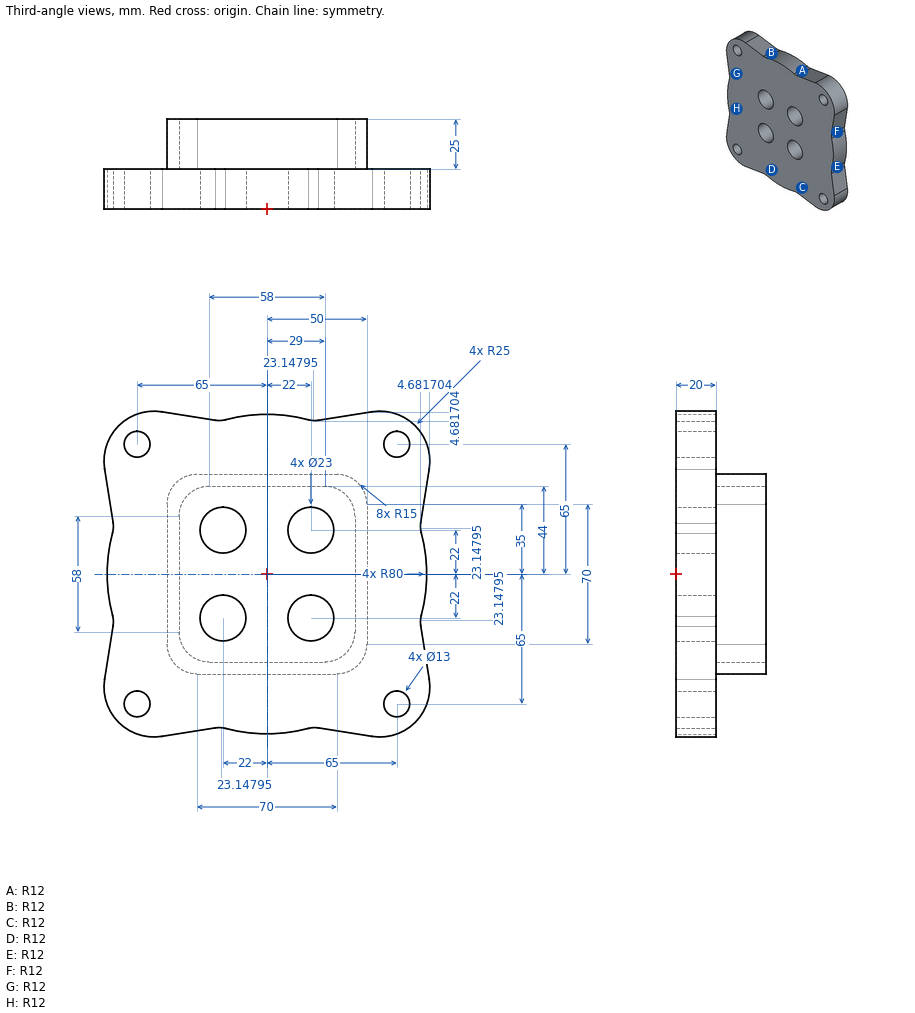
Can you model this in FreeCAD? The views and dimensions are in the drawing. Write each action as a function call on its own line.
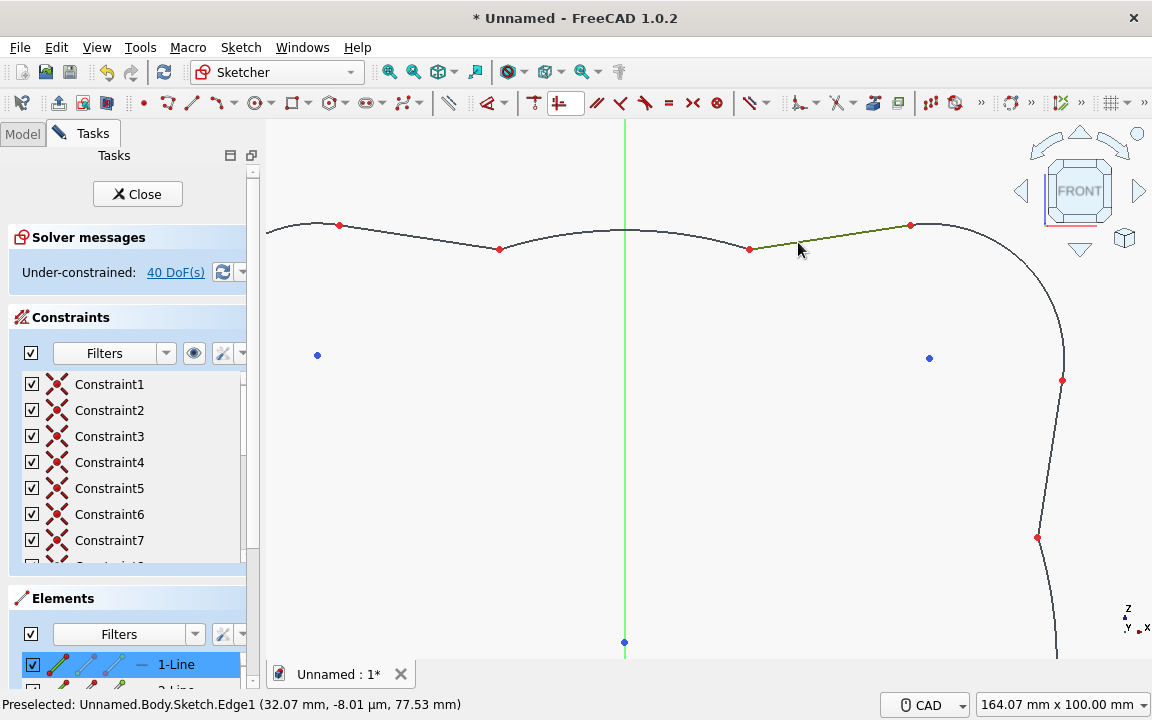
click(984, 236)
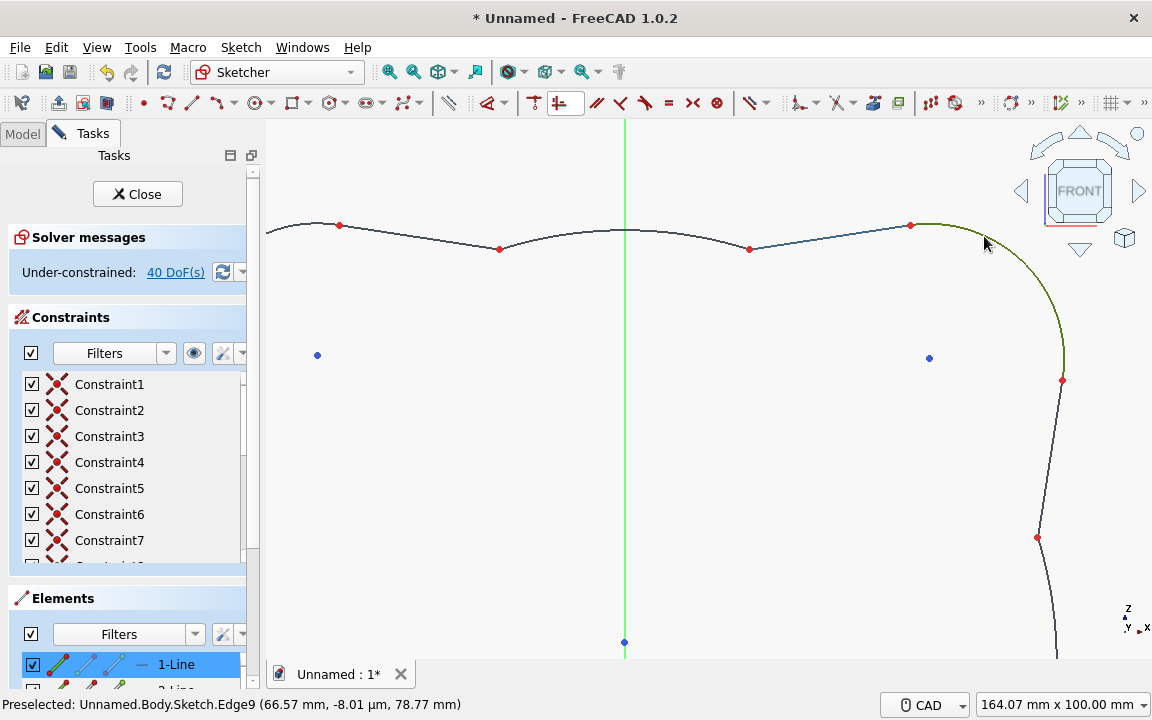
click(646, 104)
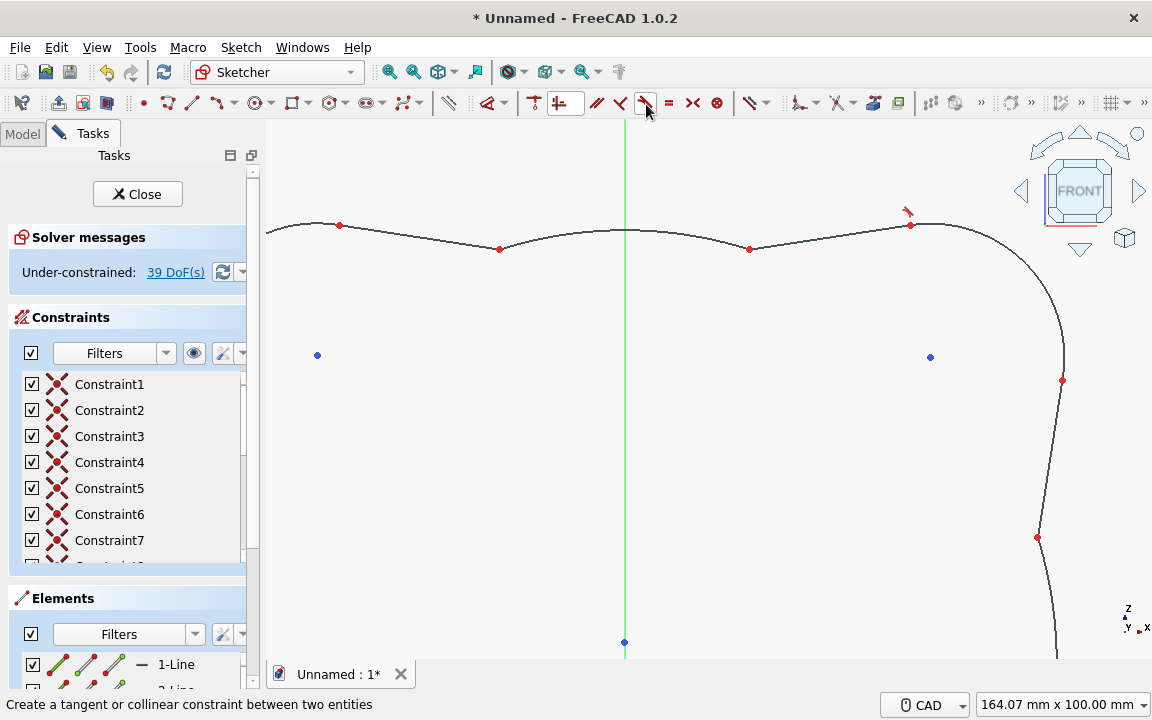
scroll(650, 231, down, 5)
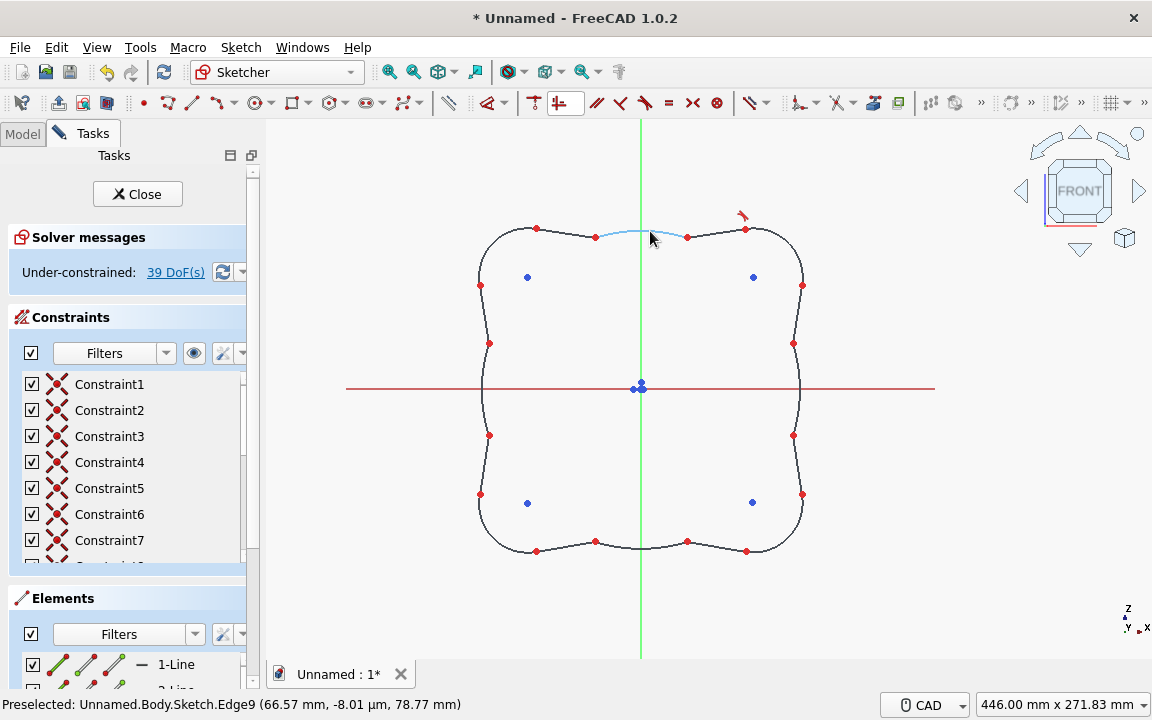
click(799, 303)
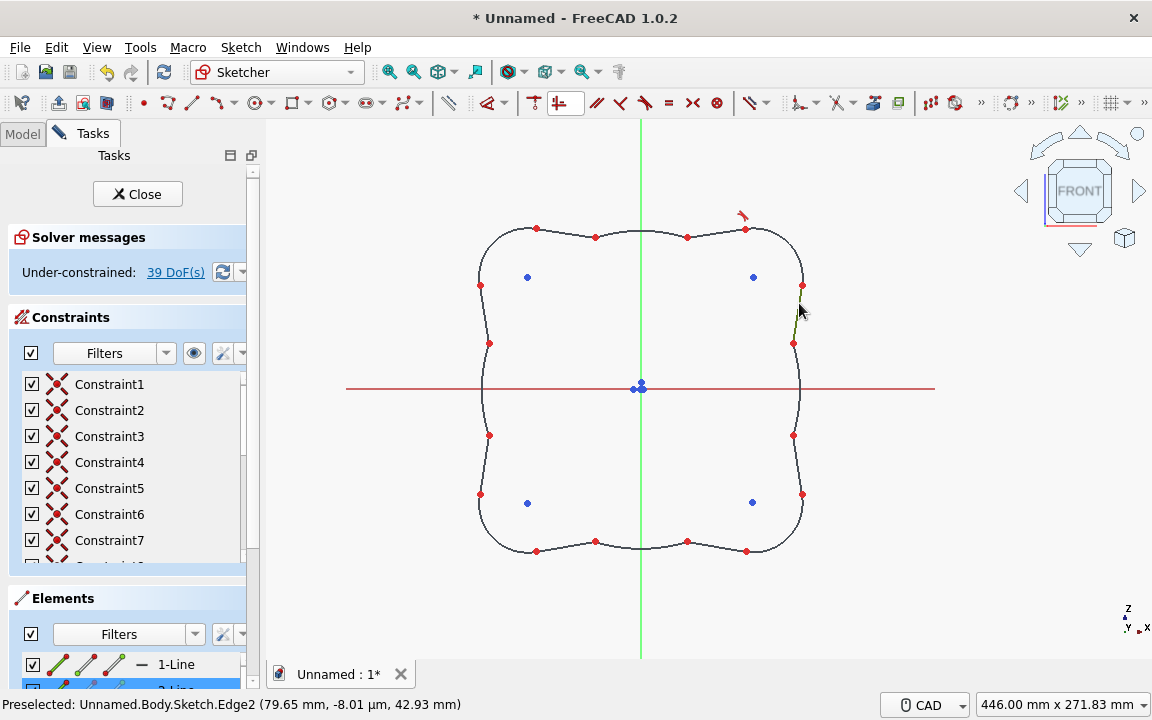
click(799, 259)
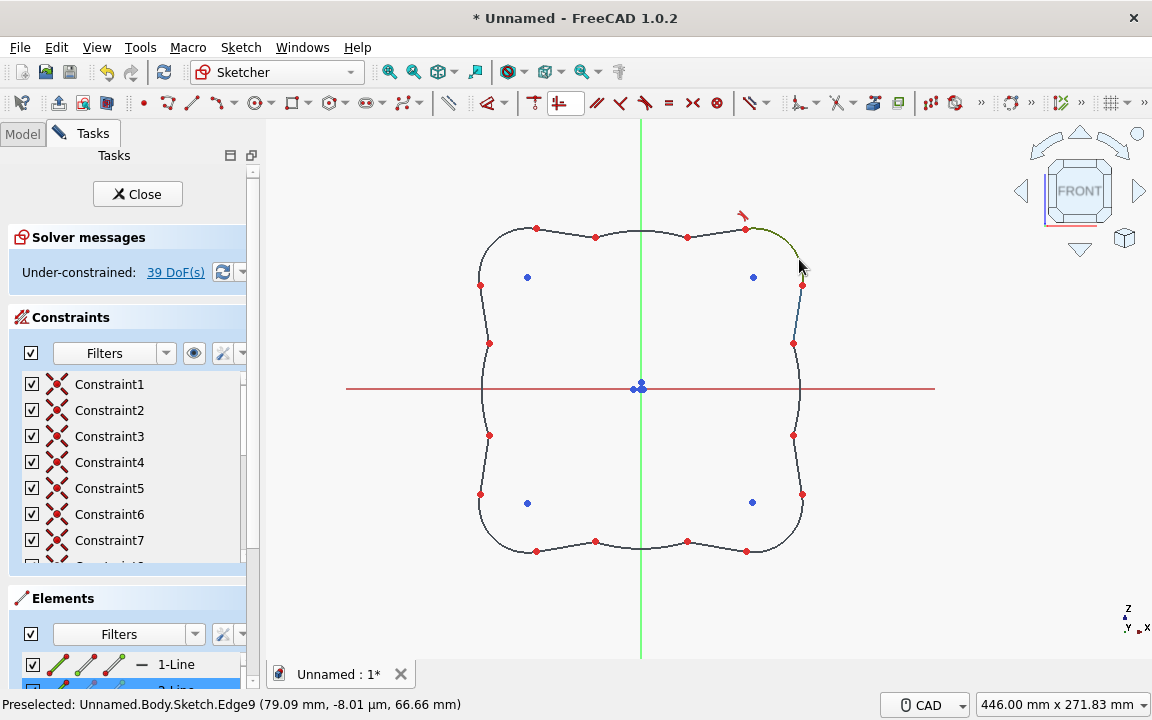
click(646, 104)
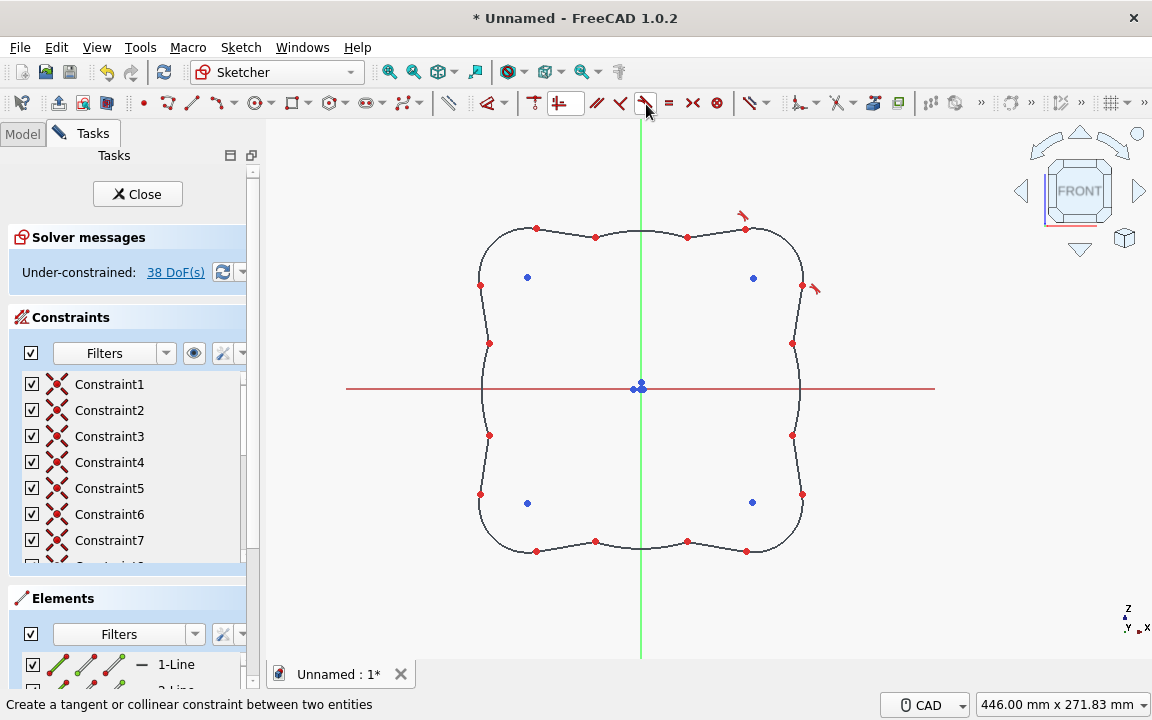
click(796, 454)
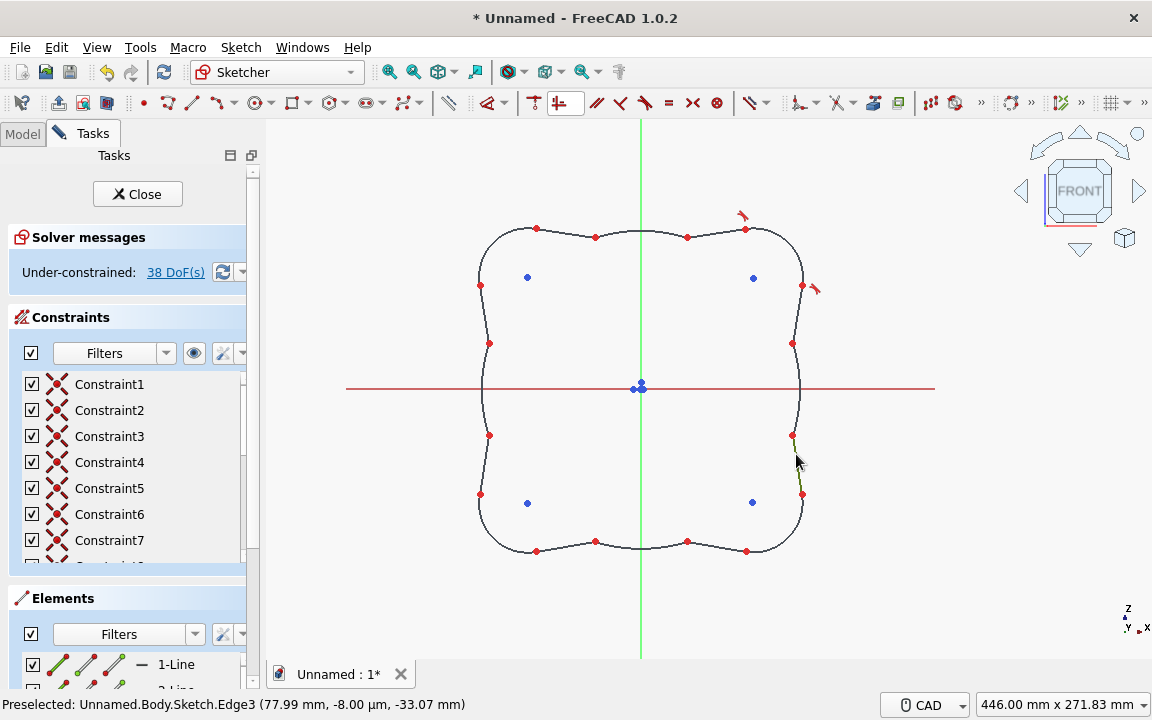
click(773, 548)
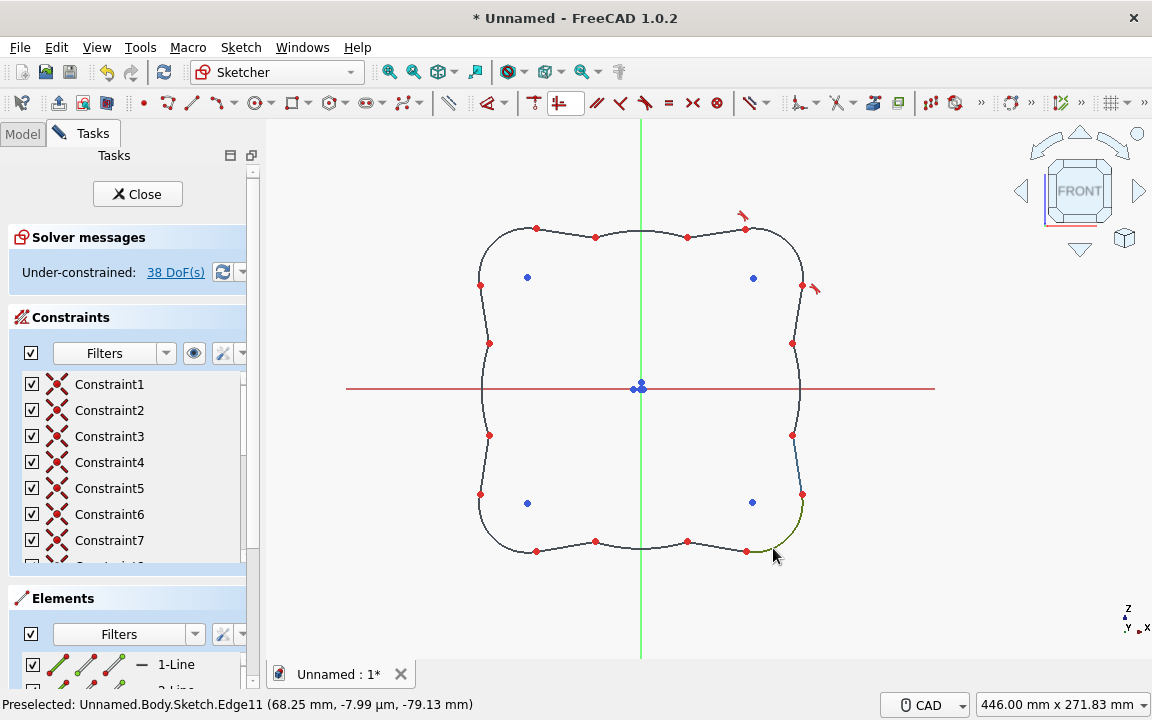
click(646, 104)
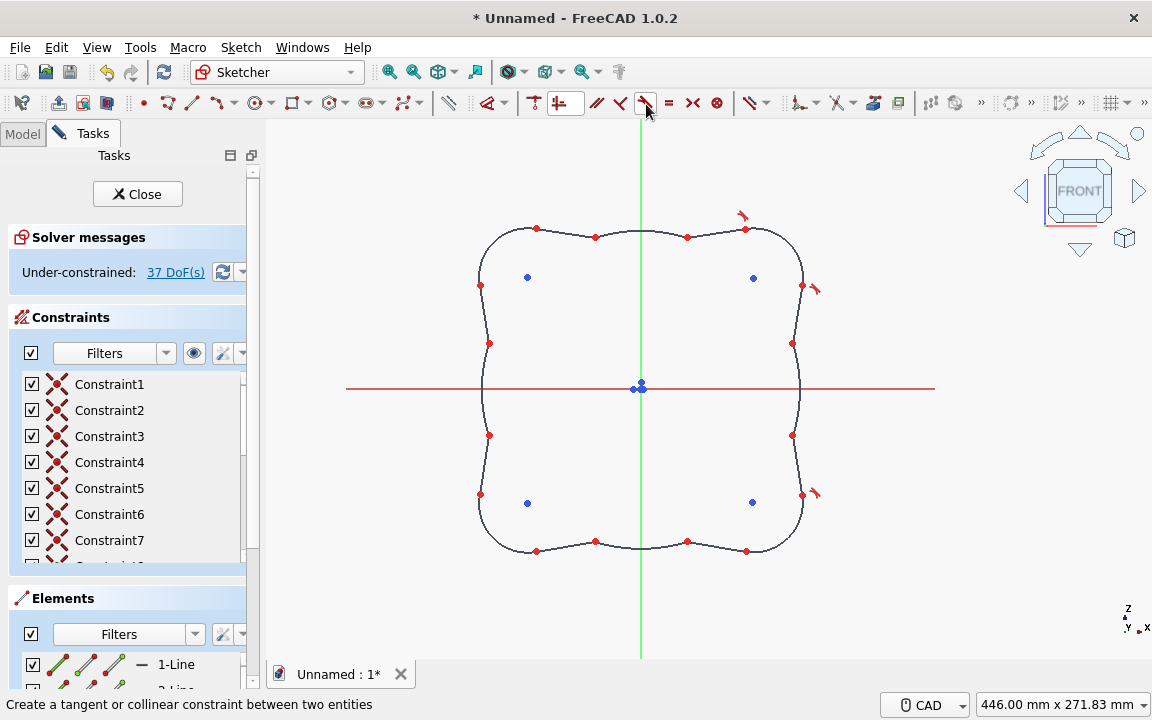
click(728, 549)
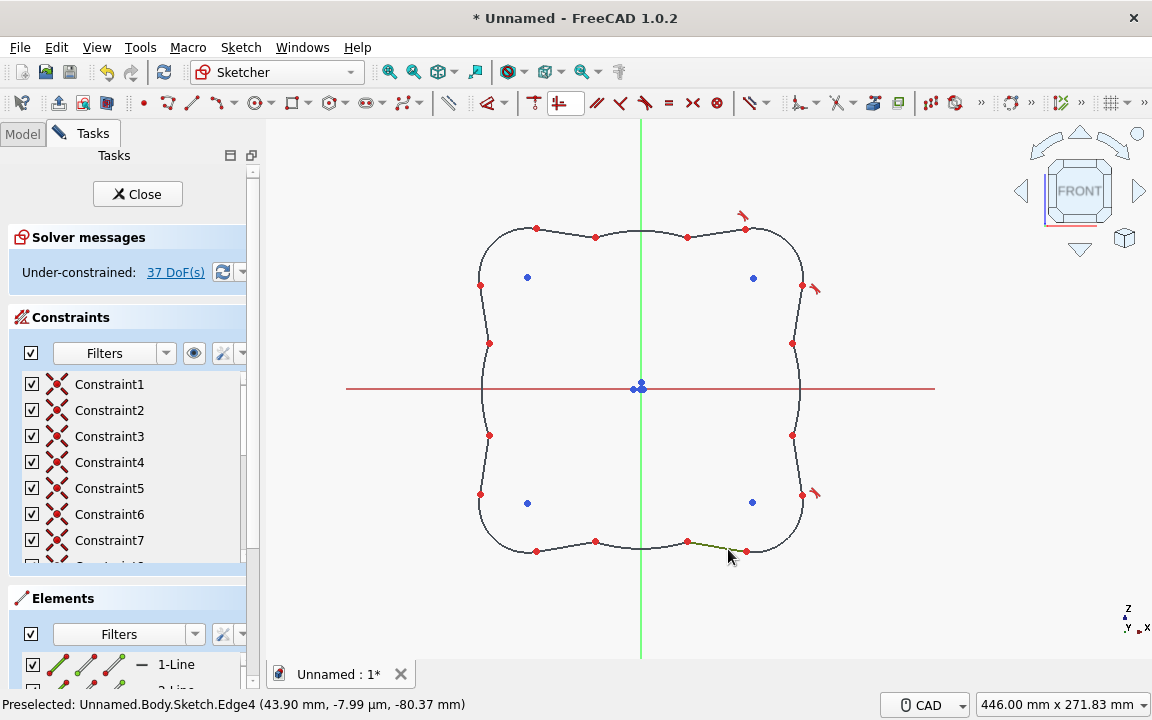
click(773, 548)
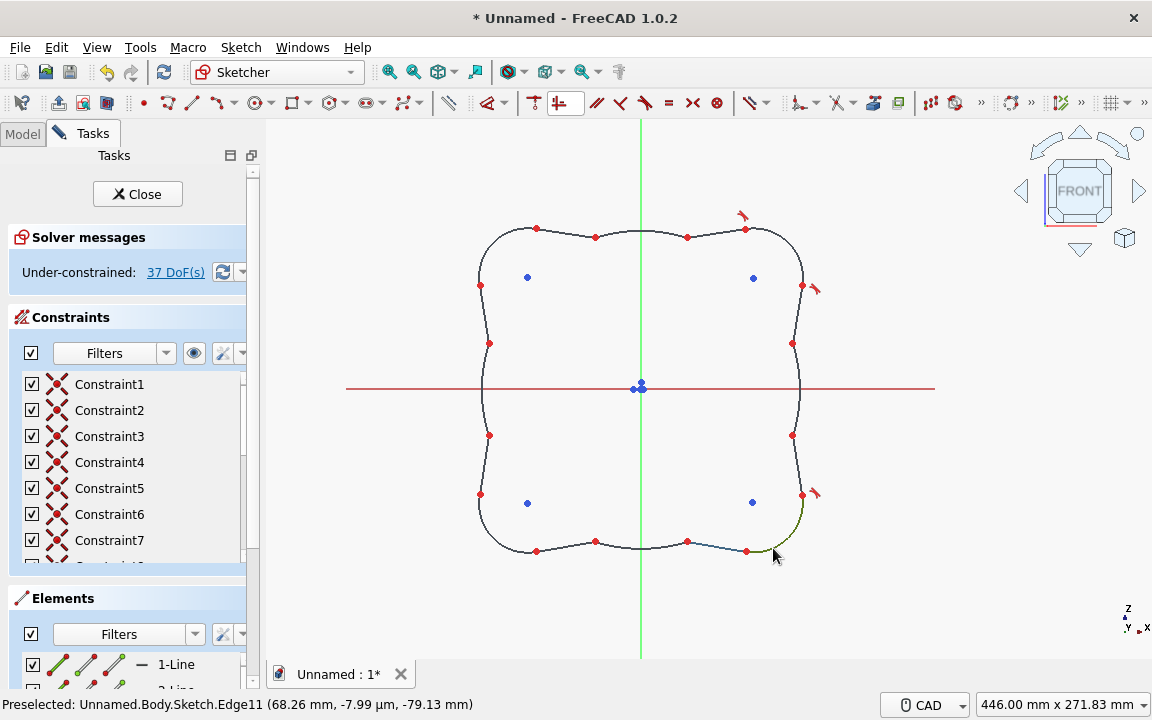
click(646, 104)